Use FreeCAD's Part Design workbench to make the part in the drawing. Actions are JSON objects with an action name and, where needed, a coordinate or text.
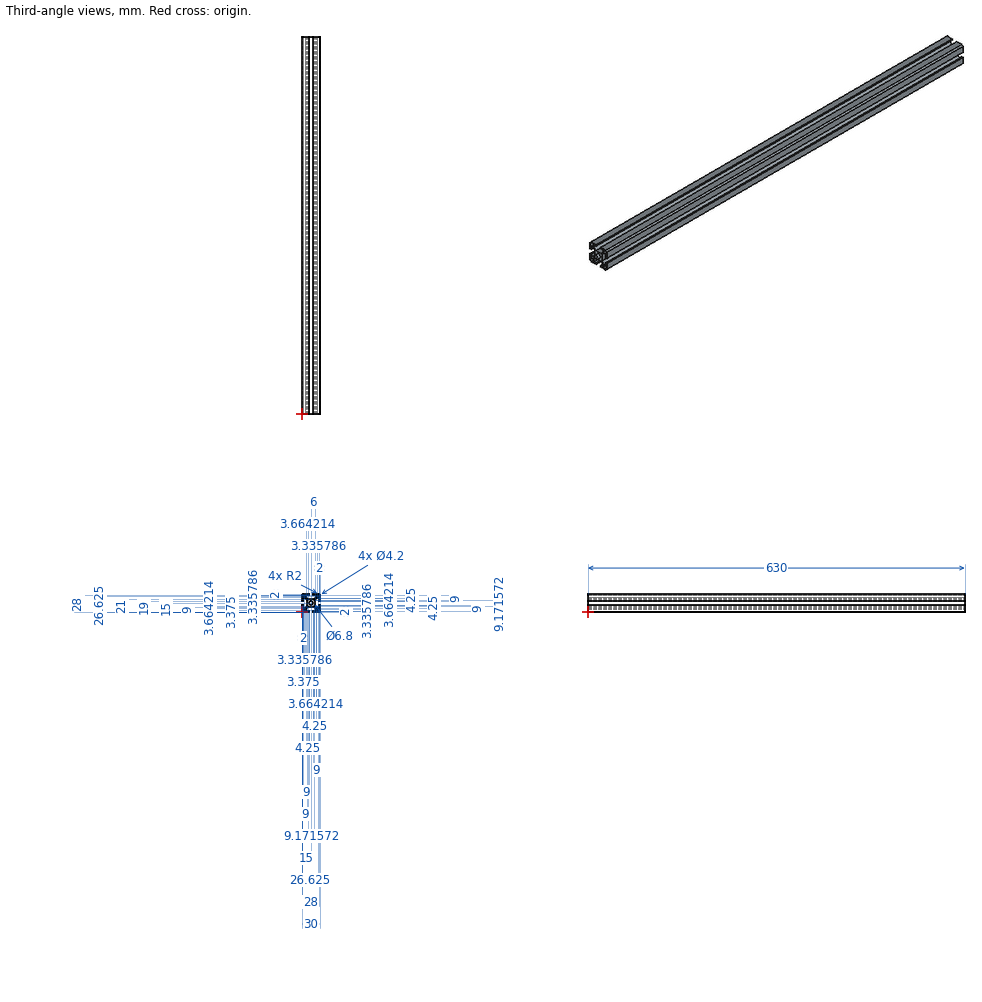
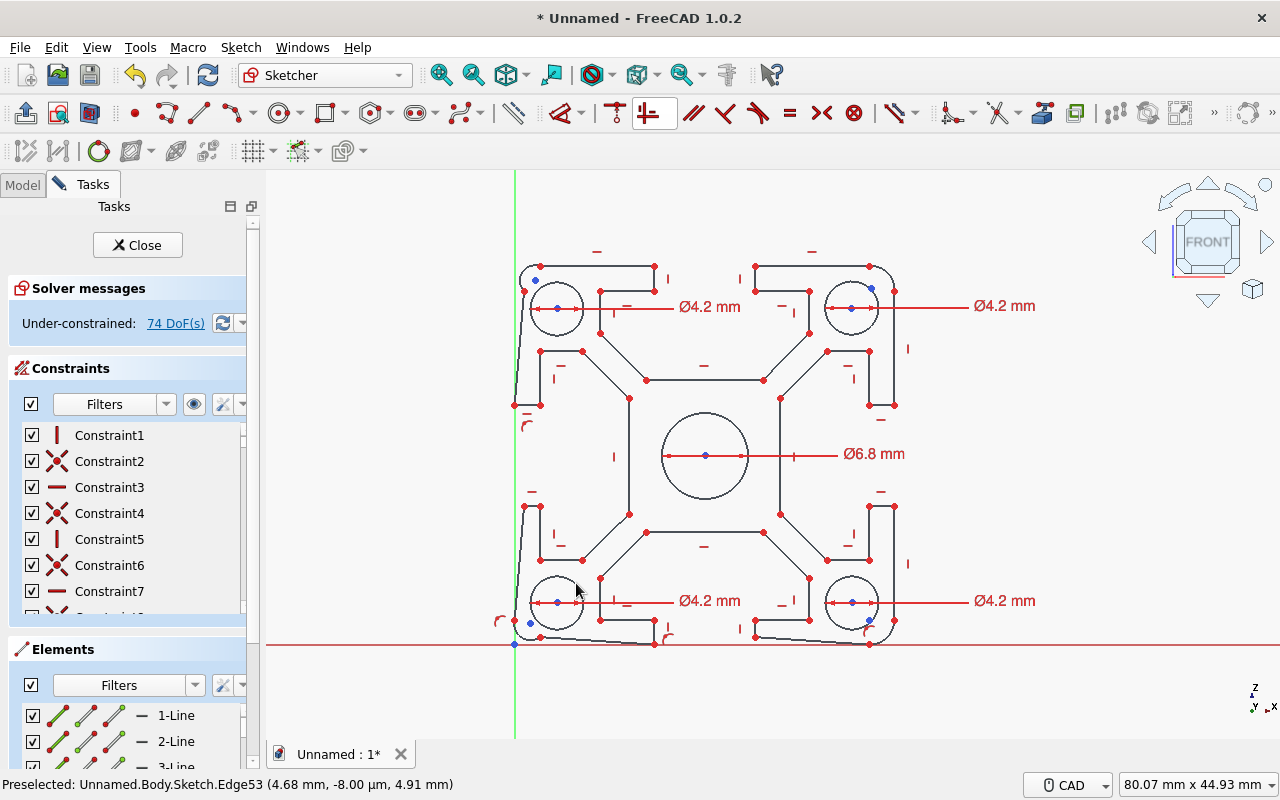
{"action": "left_click", "coordinate": [894, 325]}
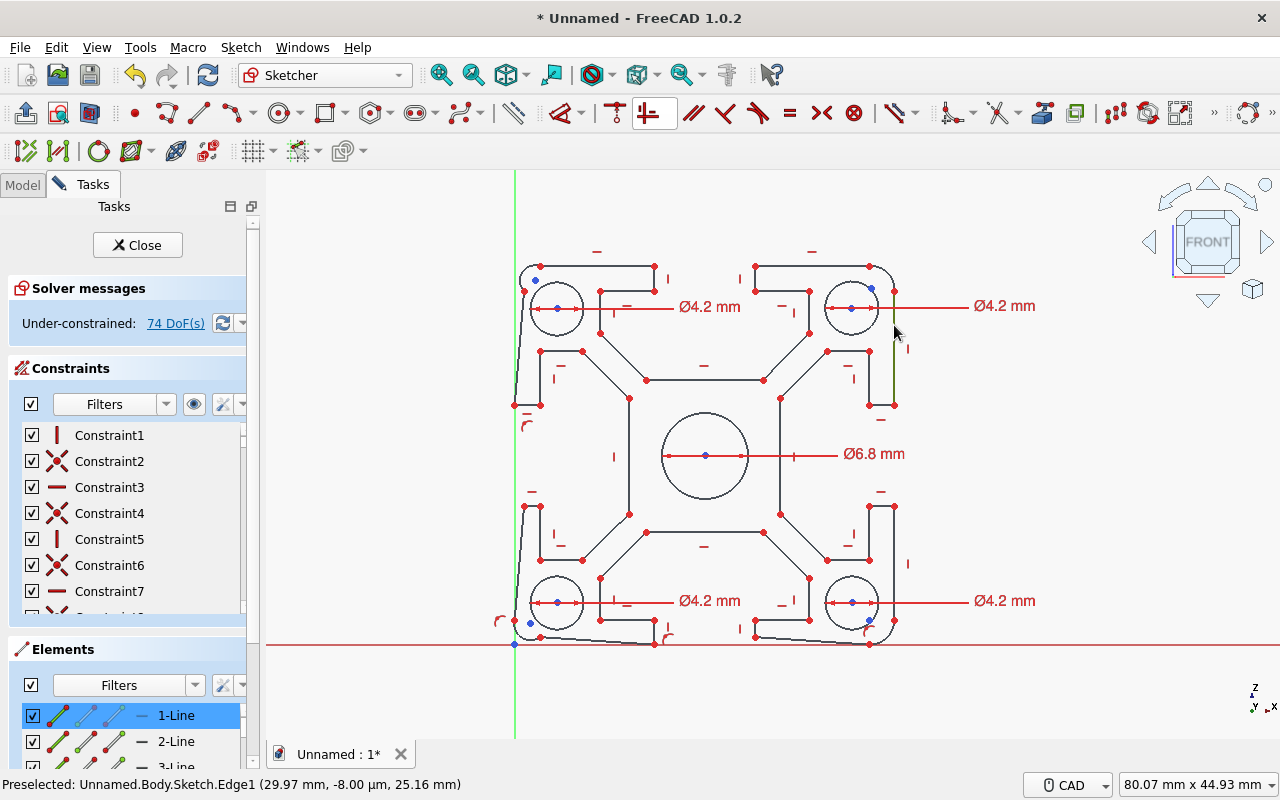
{"action": "left_click", "coordinate": [892, 279]}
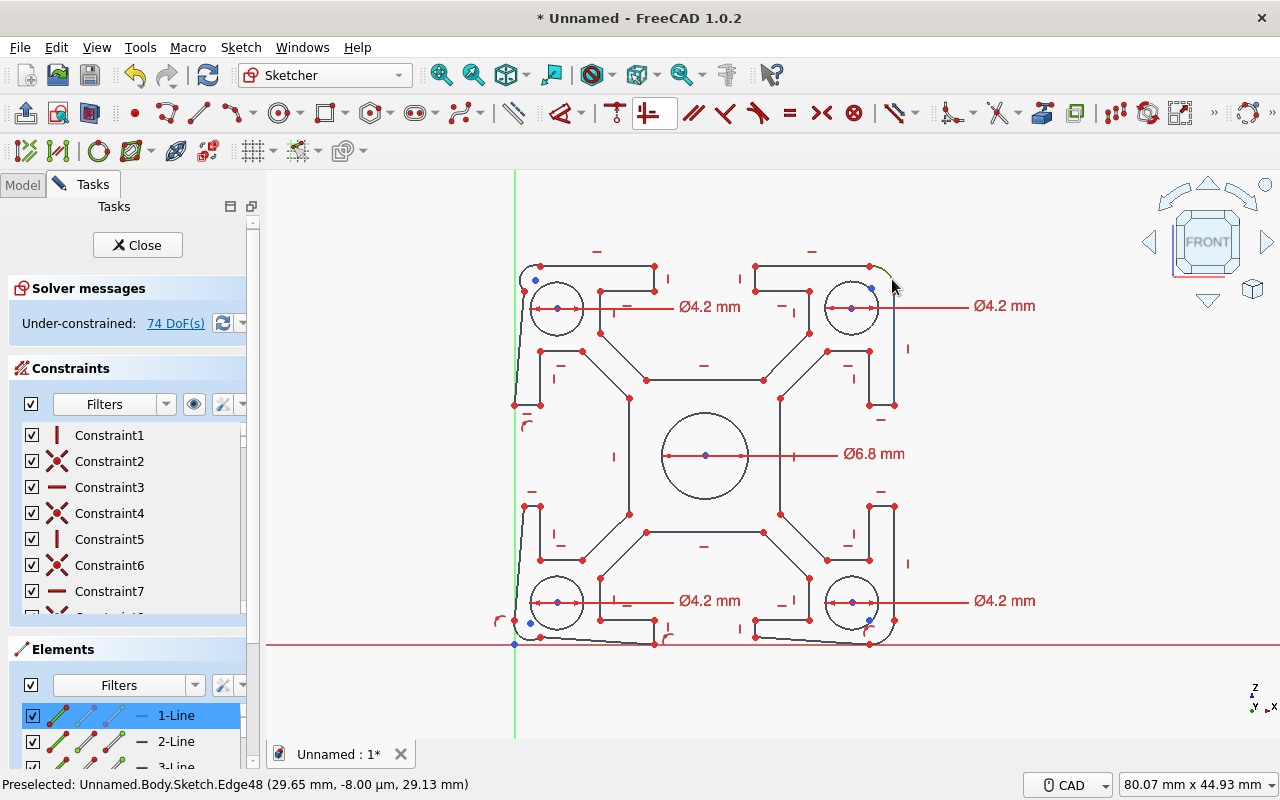
{"action": "left_click", "coordinate": [758, 114]}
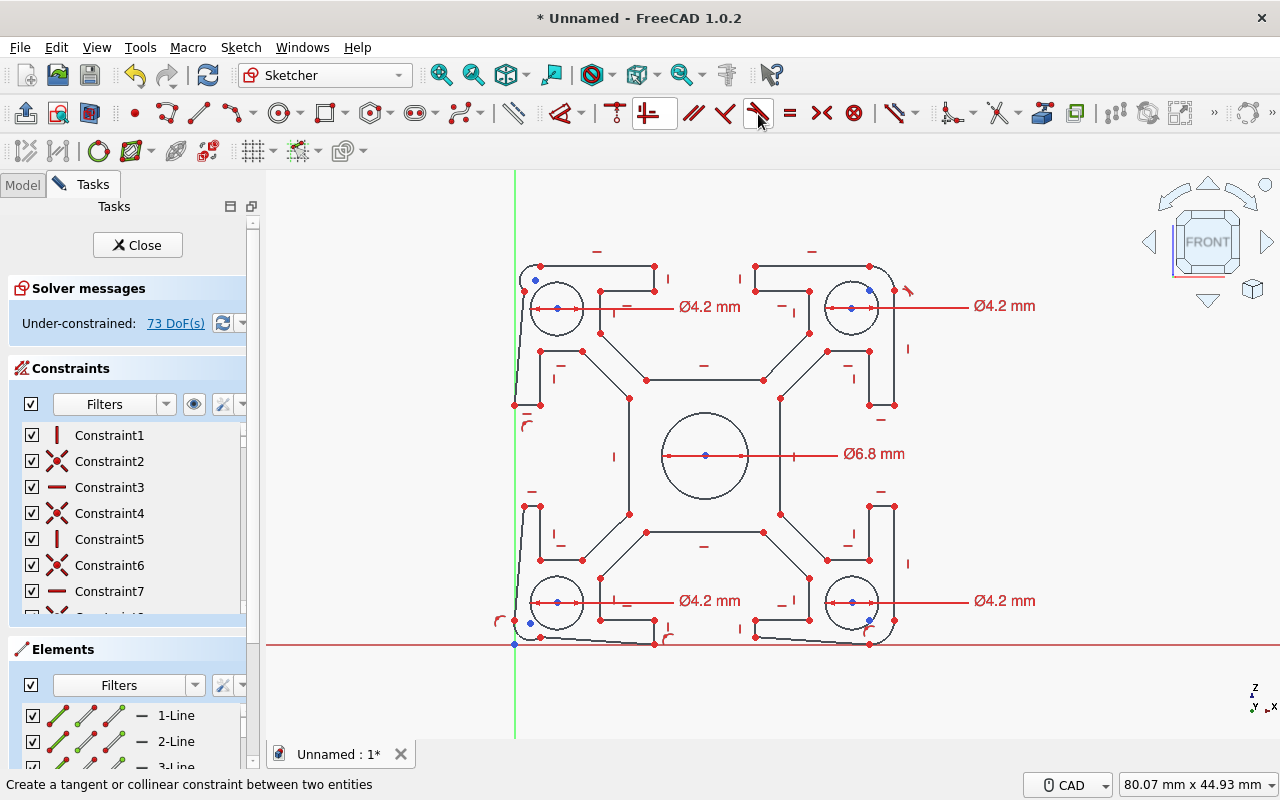
{"action": "left_click", "coordinate": [894, 540]}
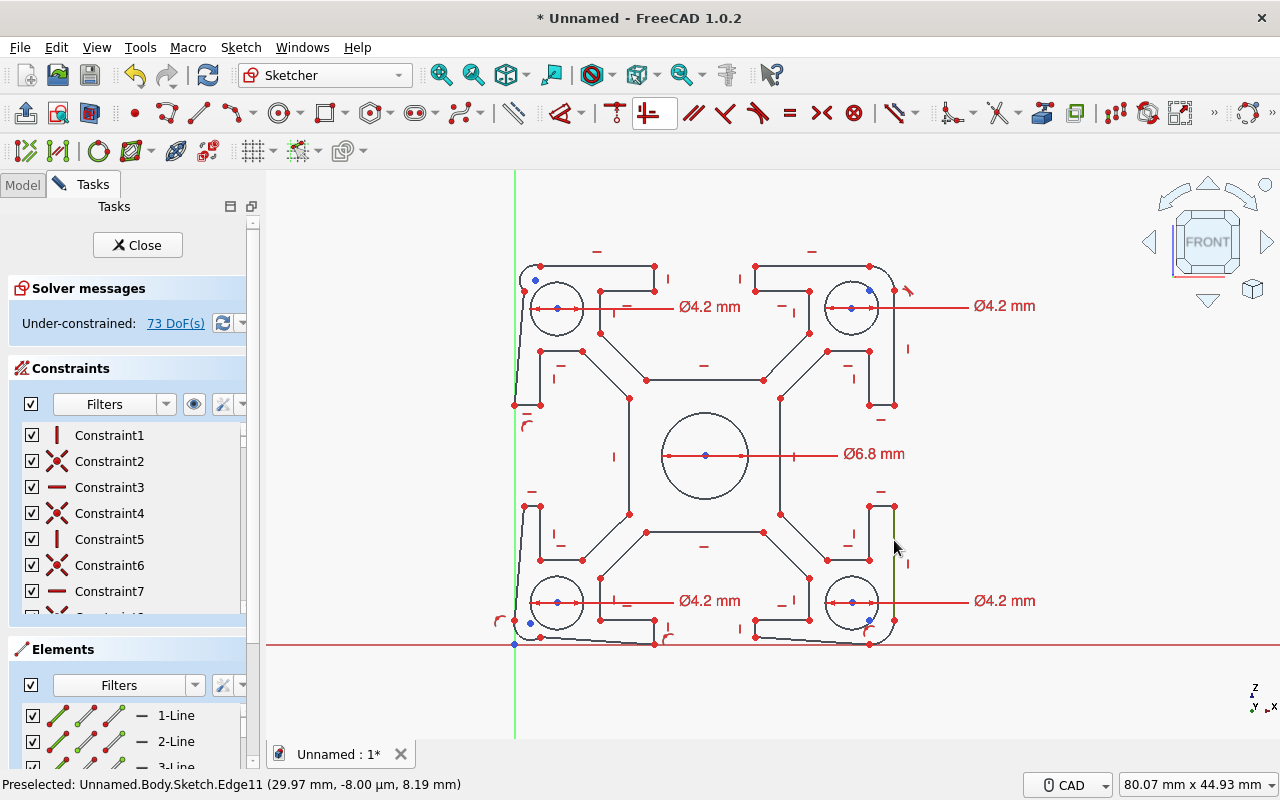
{"action": "left_click", "coordinate": [880, 642]}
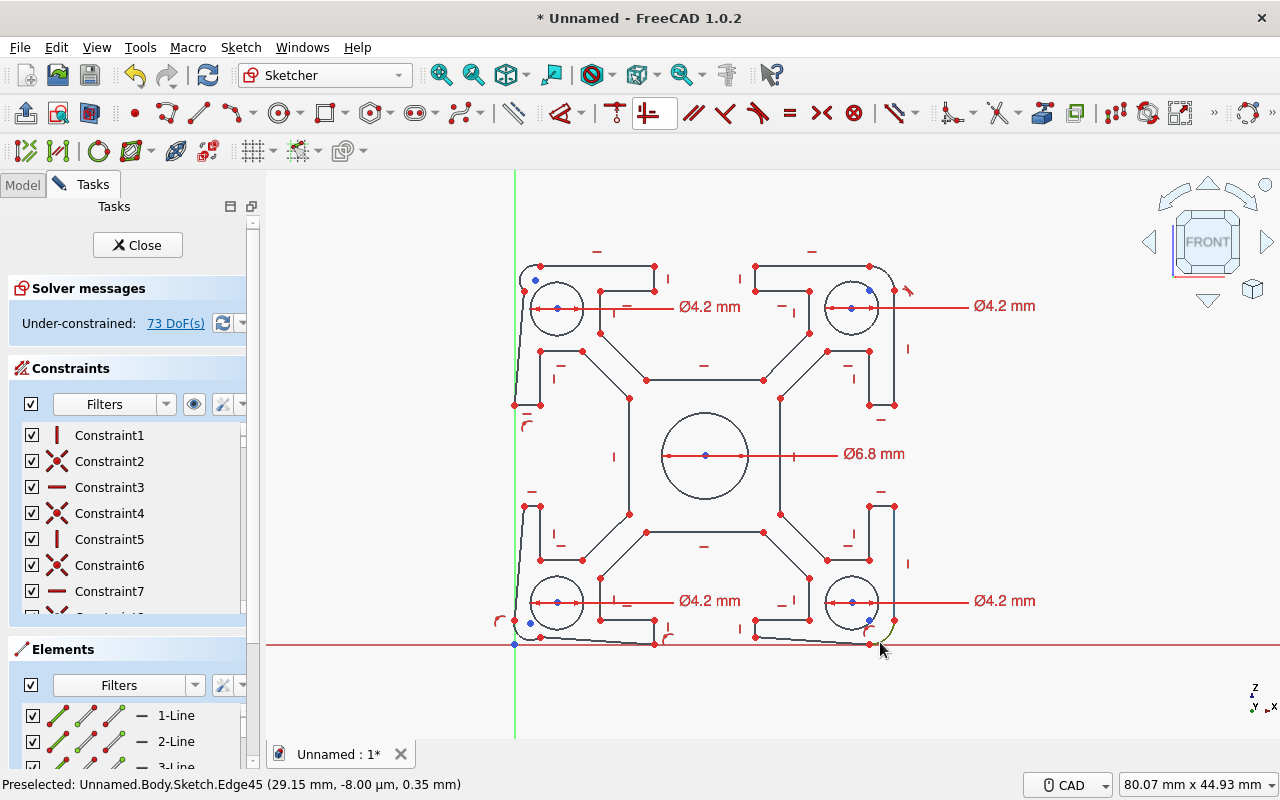
{"action": "left_click", "coordinate": [758, 114]}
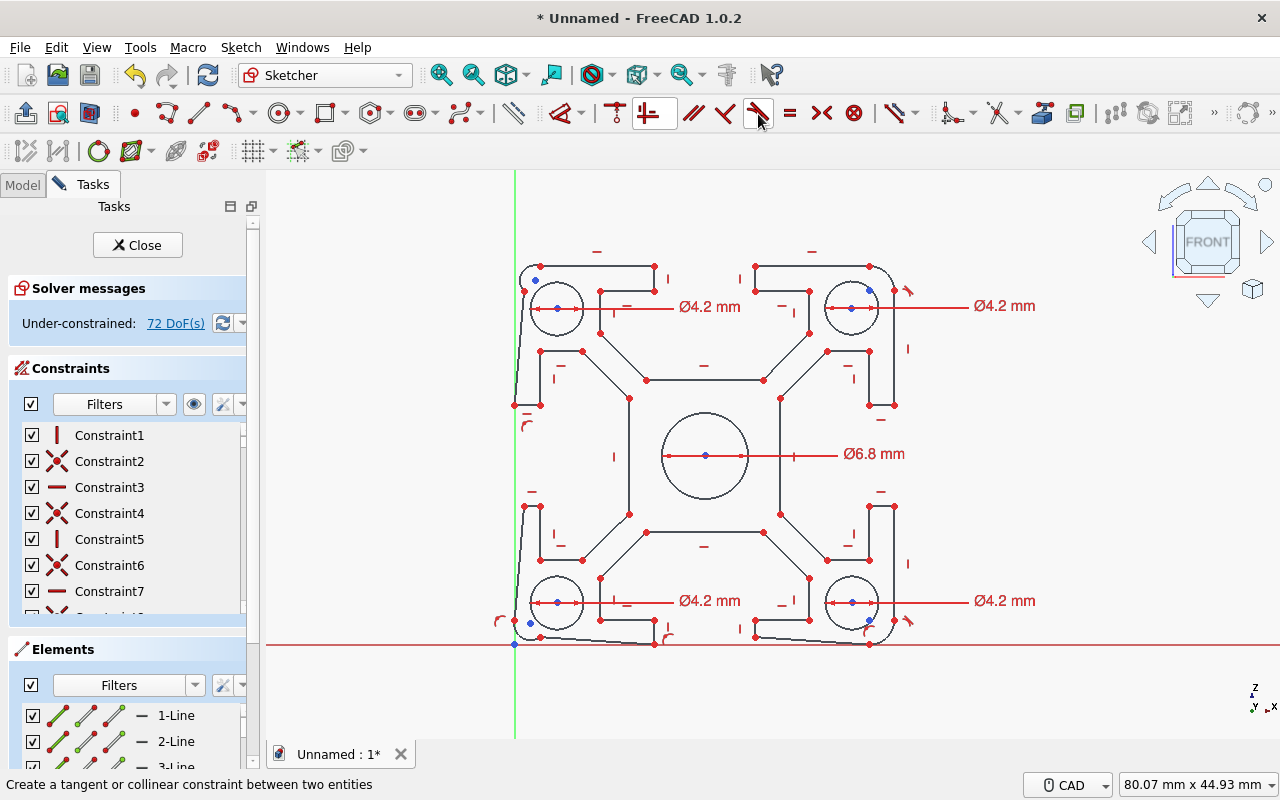
{"action": "left_click", "coordinate": [835, 642]}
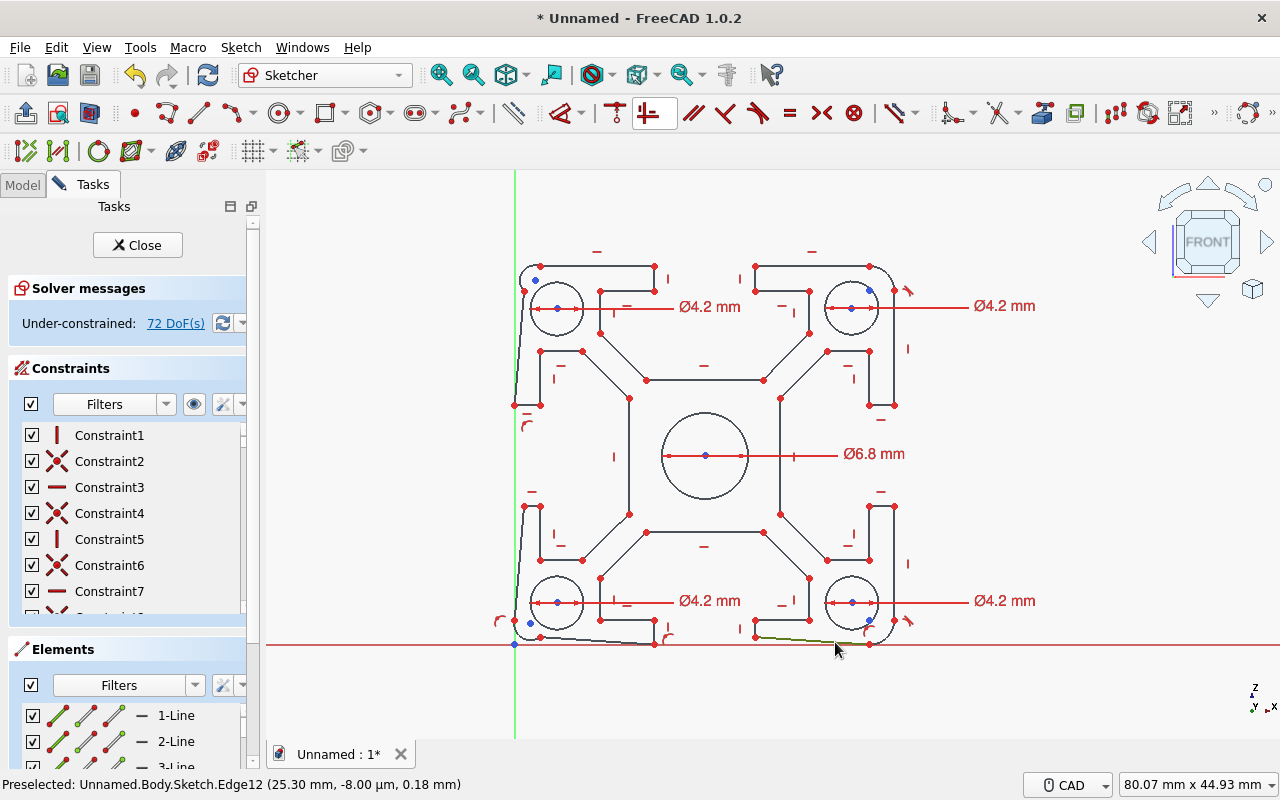
{"action": "left_click", "coordinate": [880, 642]}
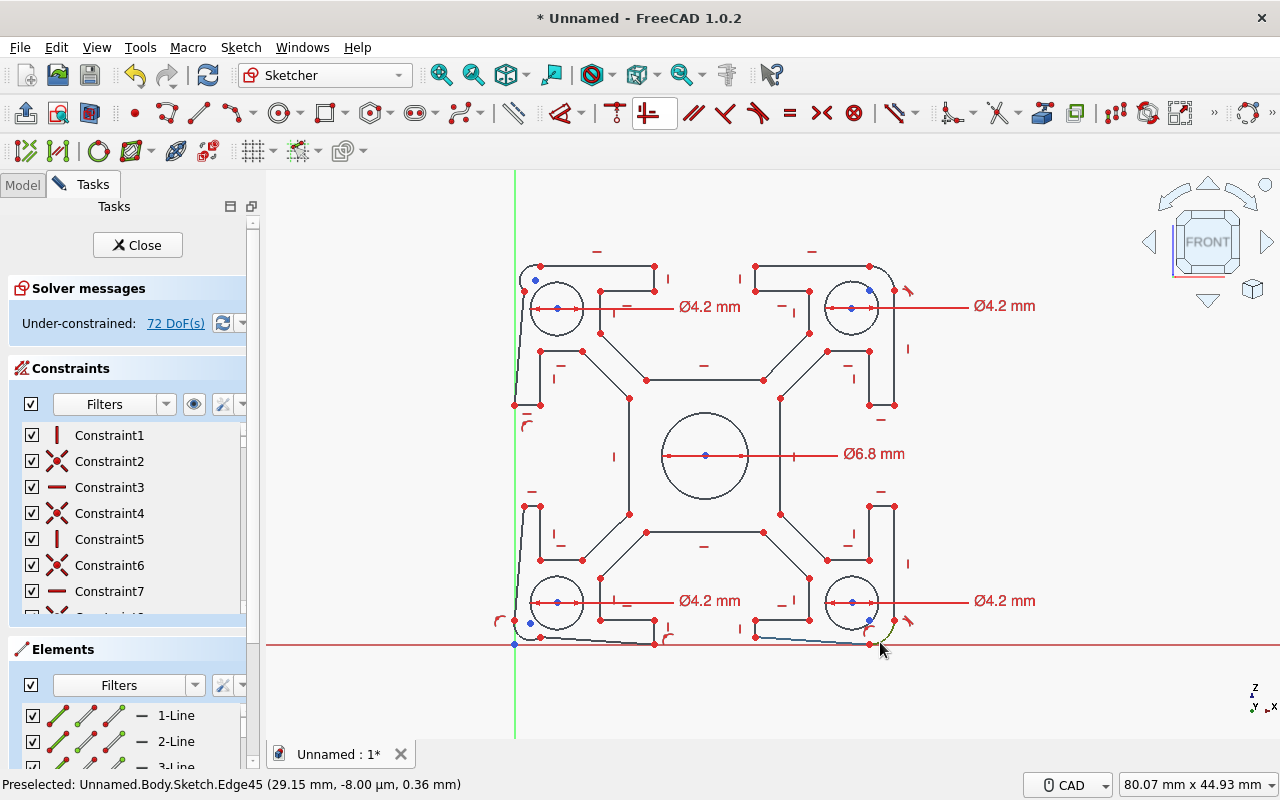
{"action": "left_click", "coordinate": [758, 114]}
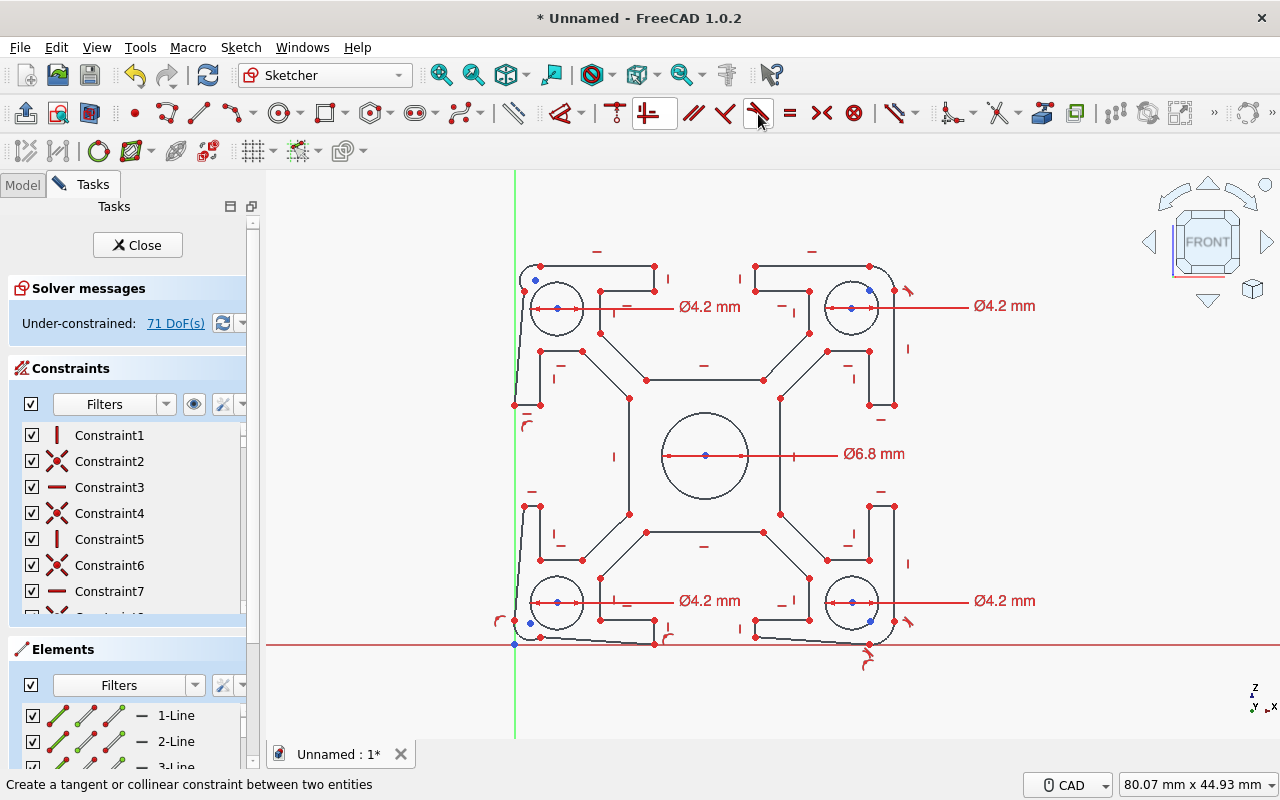
{"action": "left_click", "coordinate": [620, 642]}